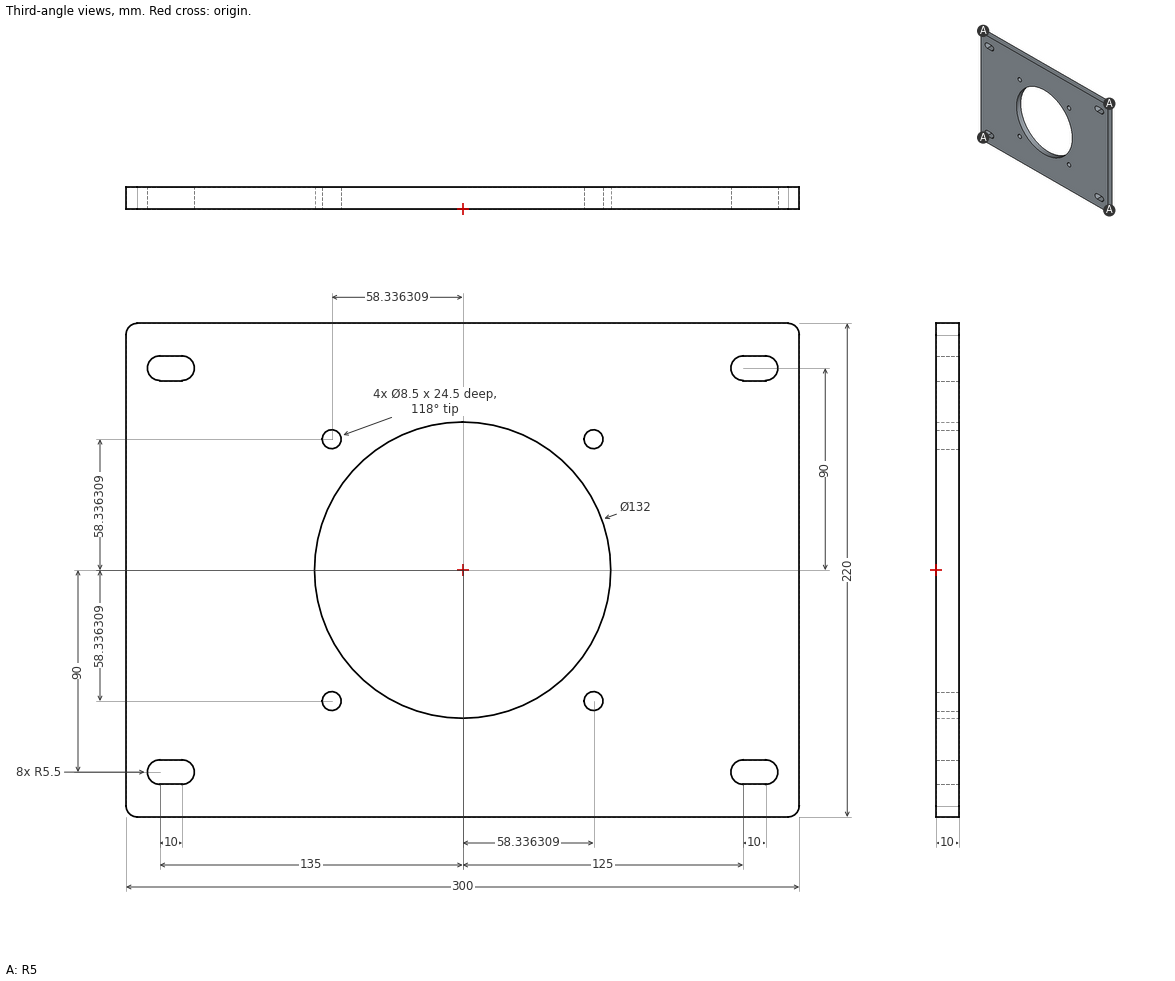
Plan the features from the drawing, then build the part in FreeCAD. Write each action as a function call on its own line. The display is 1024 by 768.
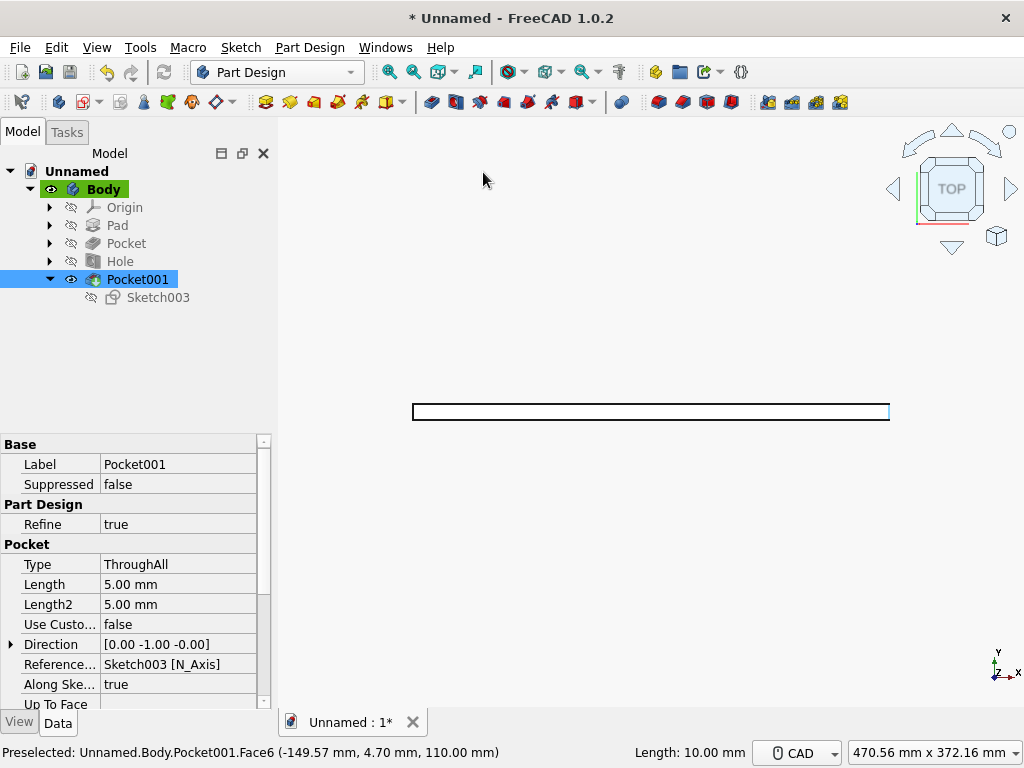
click(413, 411, ctrl)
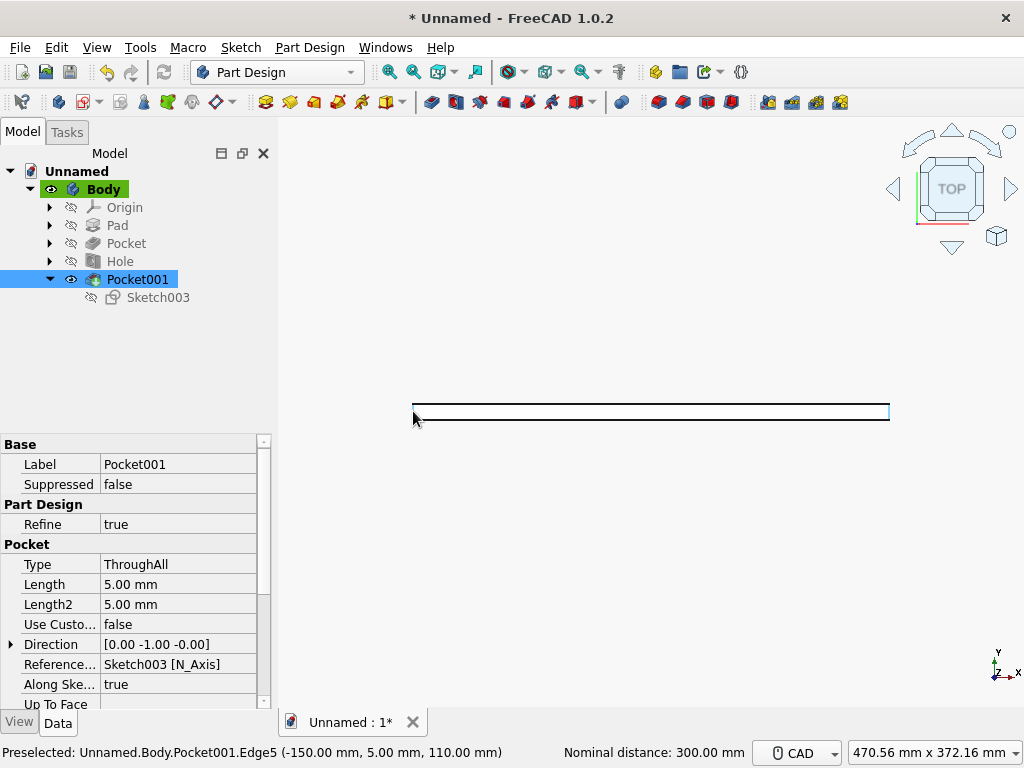
scroll(413, 411, up, 5)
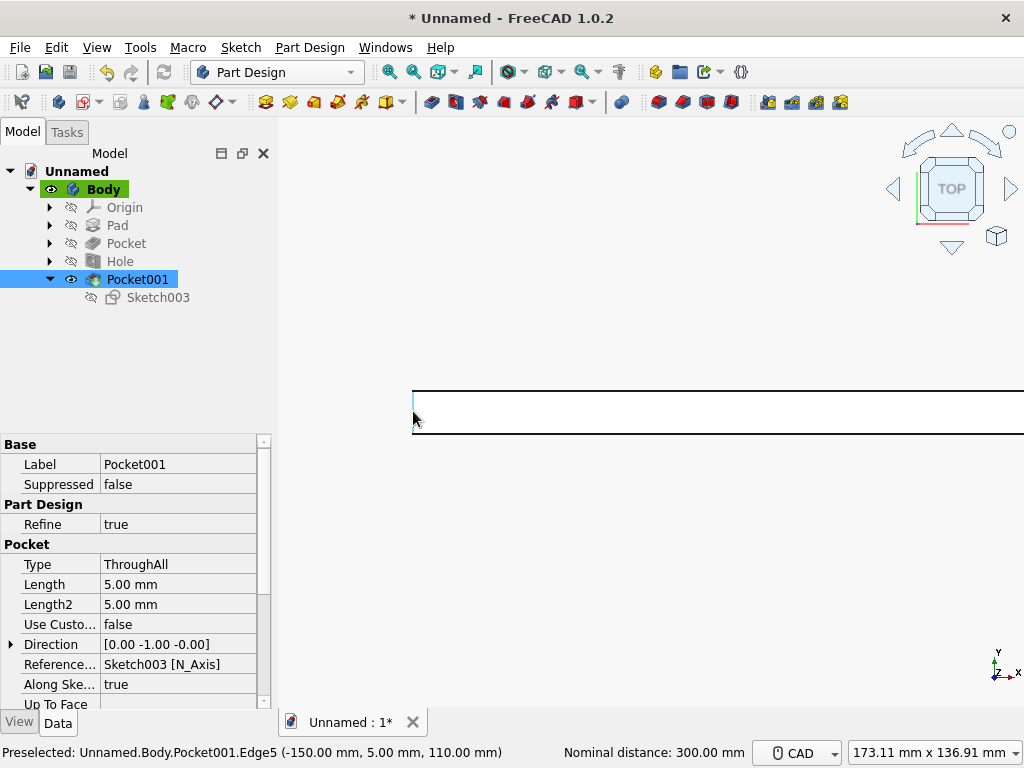
key(v)
key(f)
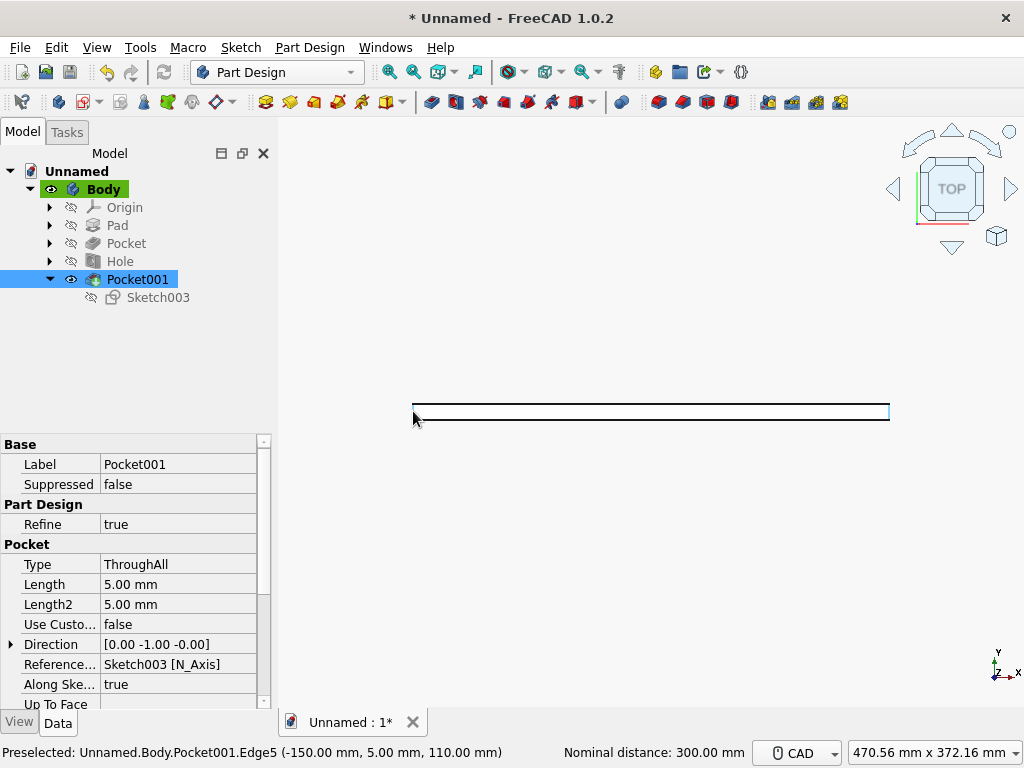
key(1)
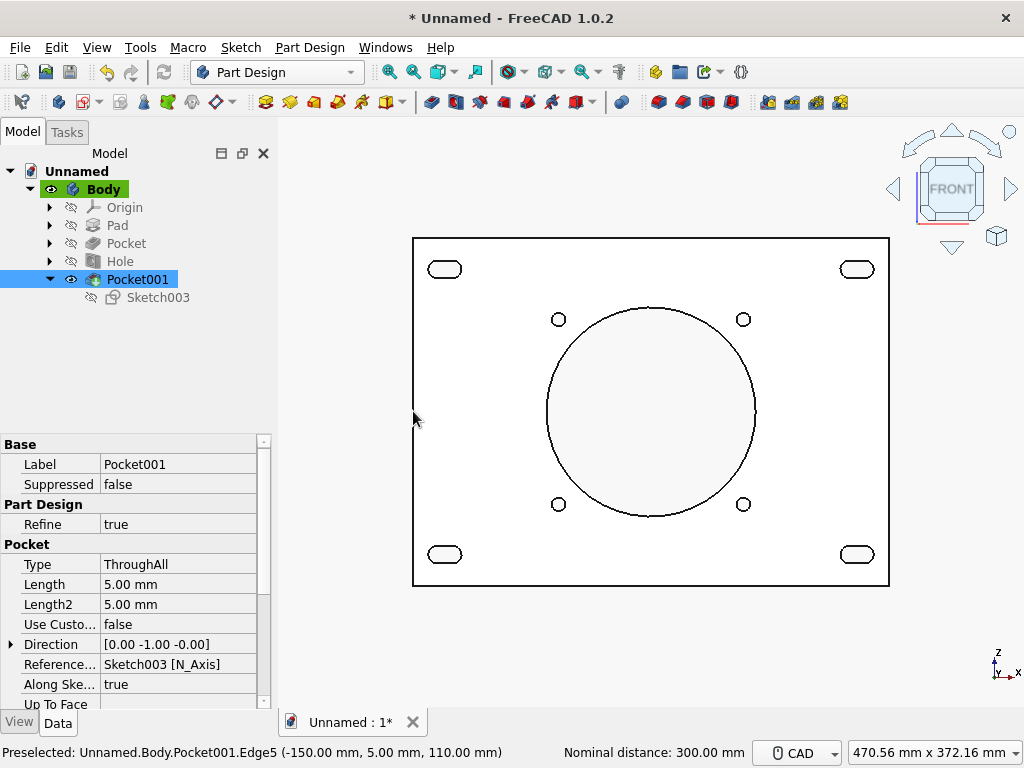
scroll(413, 585, up, 5)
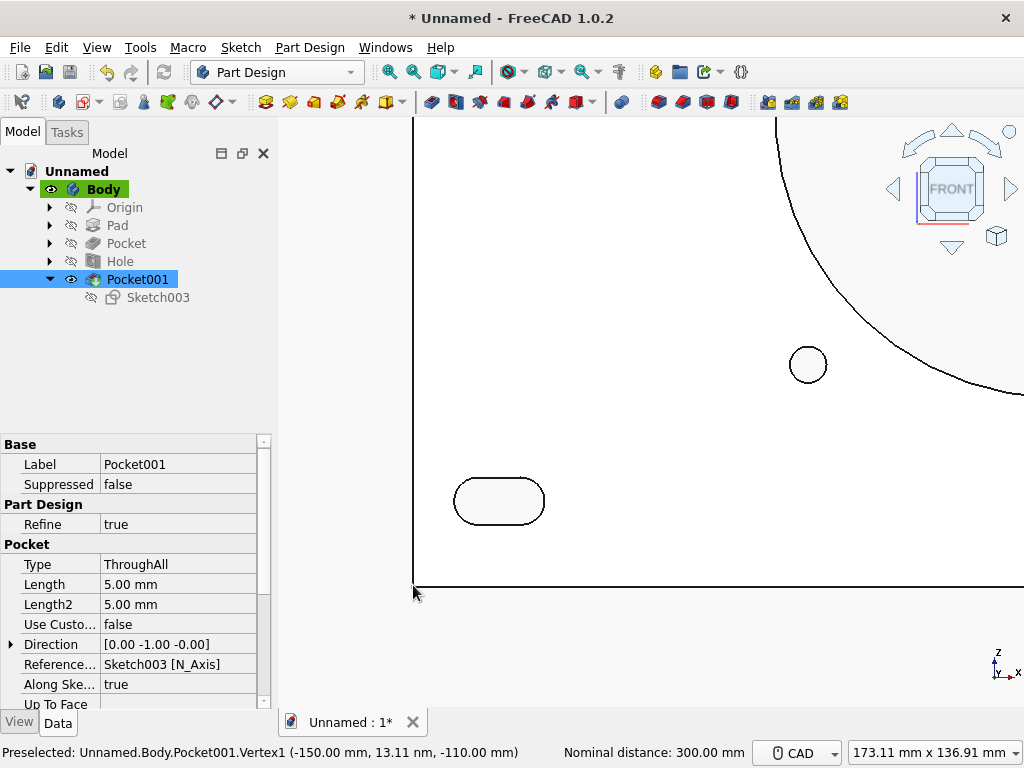
click(390, 72)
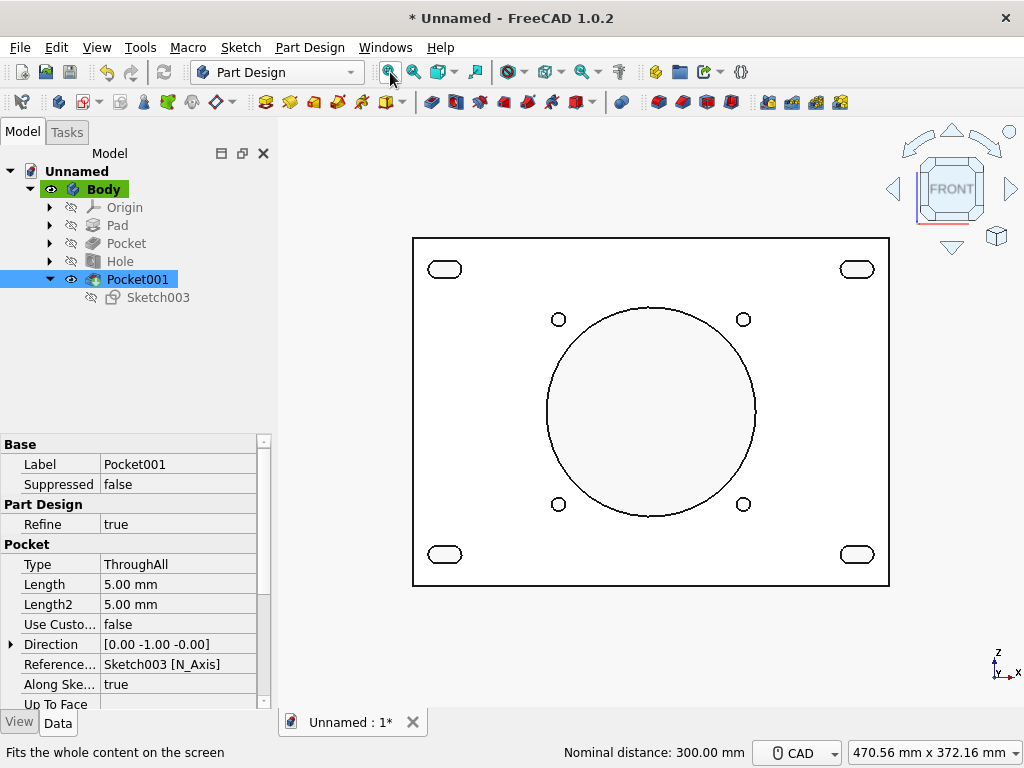
key(3)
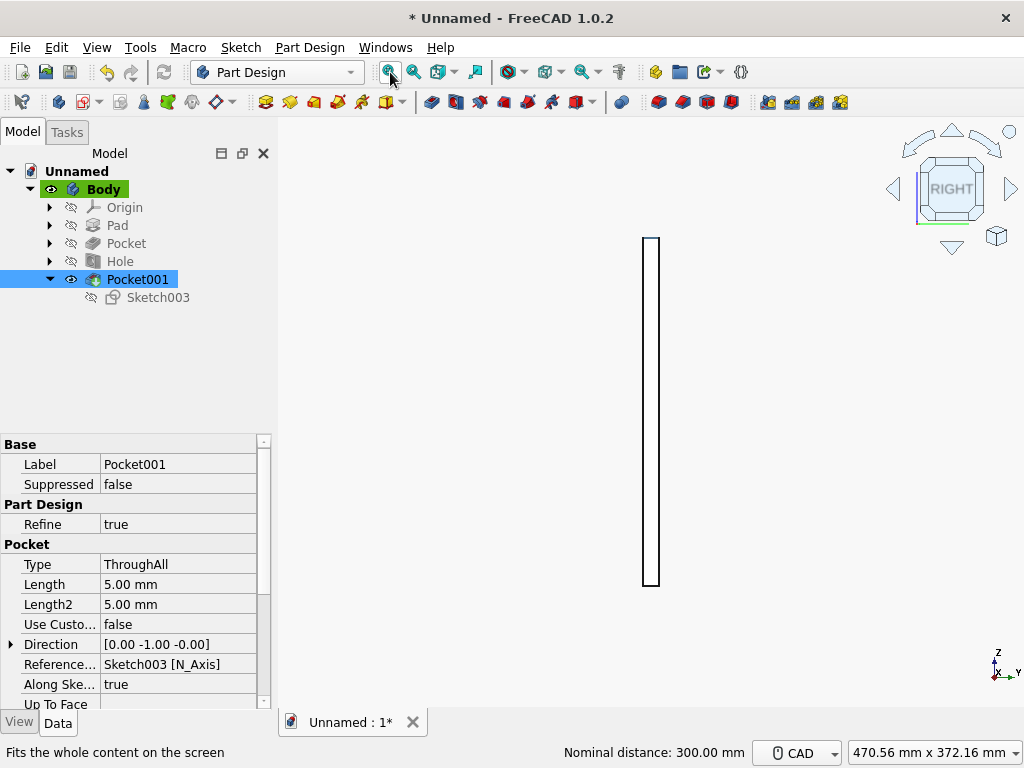
click(651, 585, ctrl)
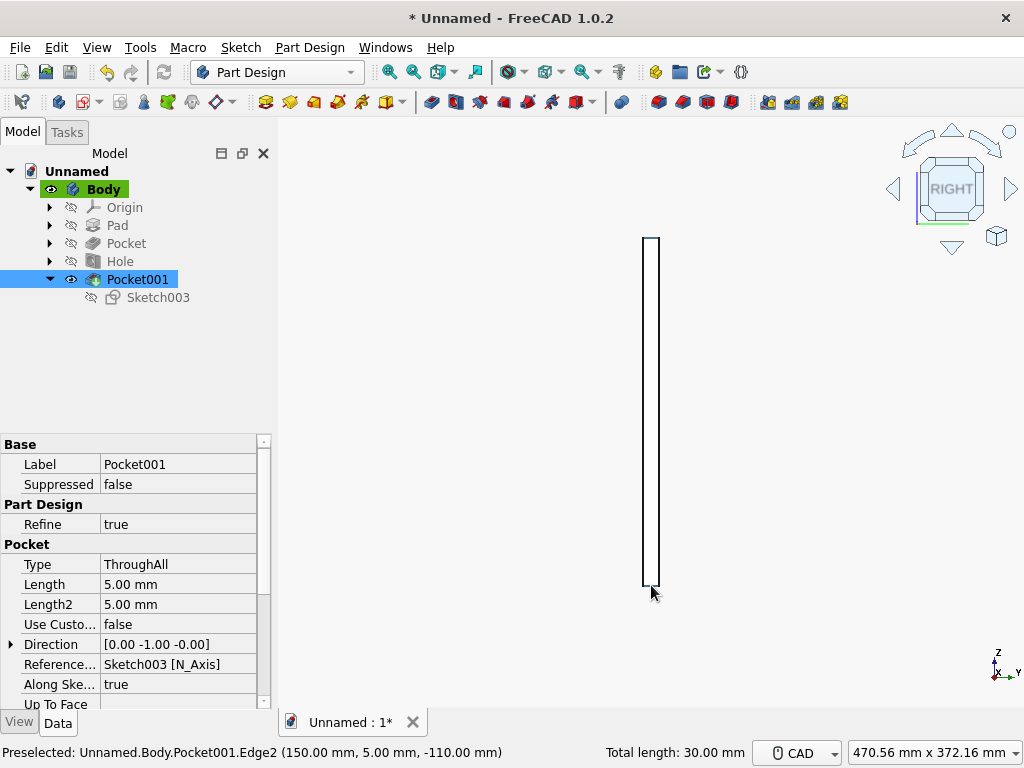
scroll(651, 585, up, 5)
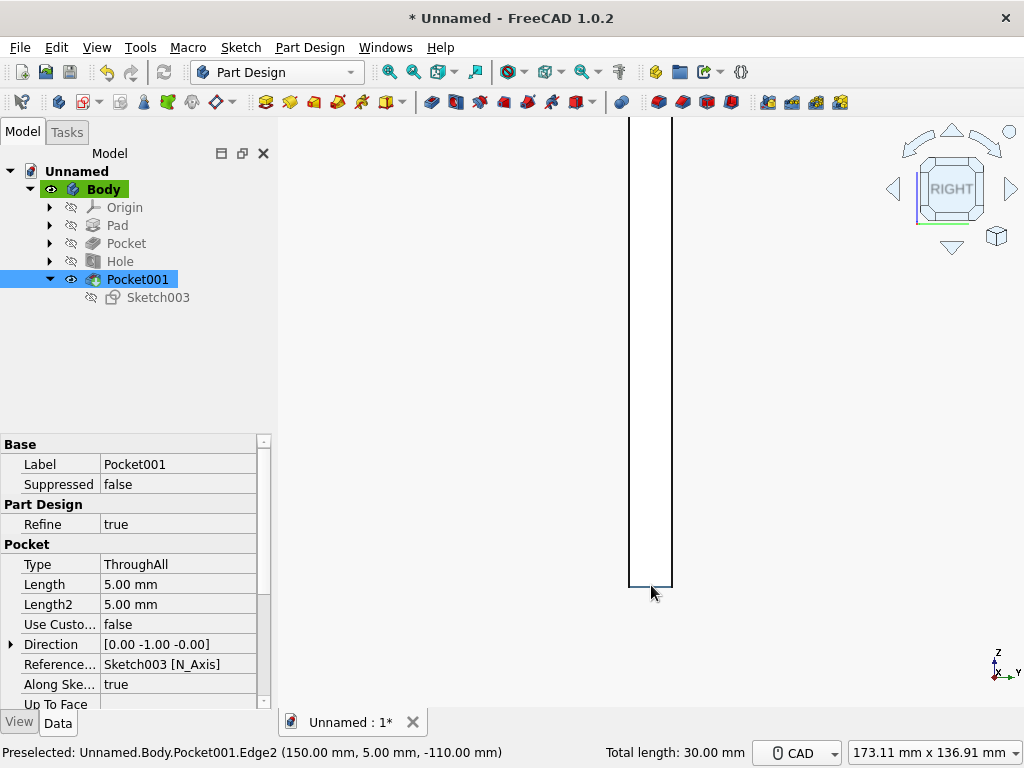
click(390, 72)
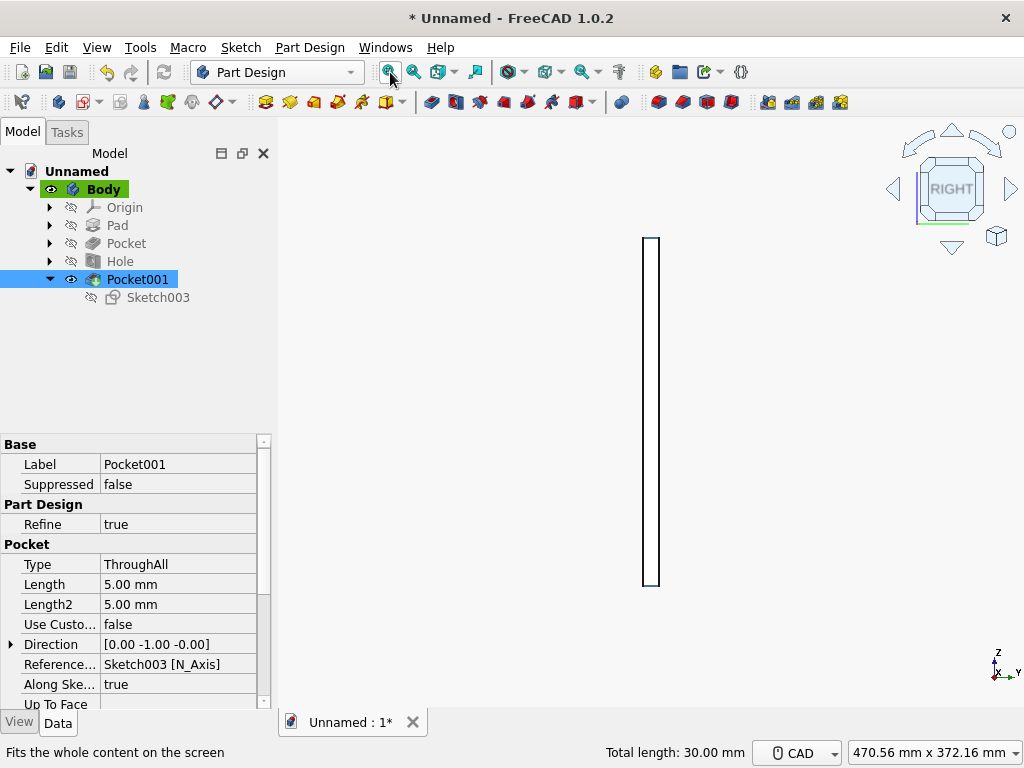
key(5)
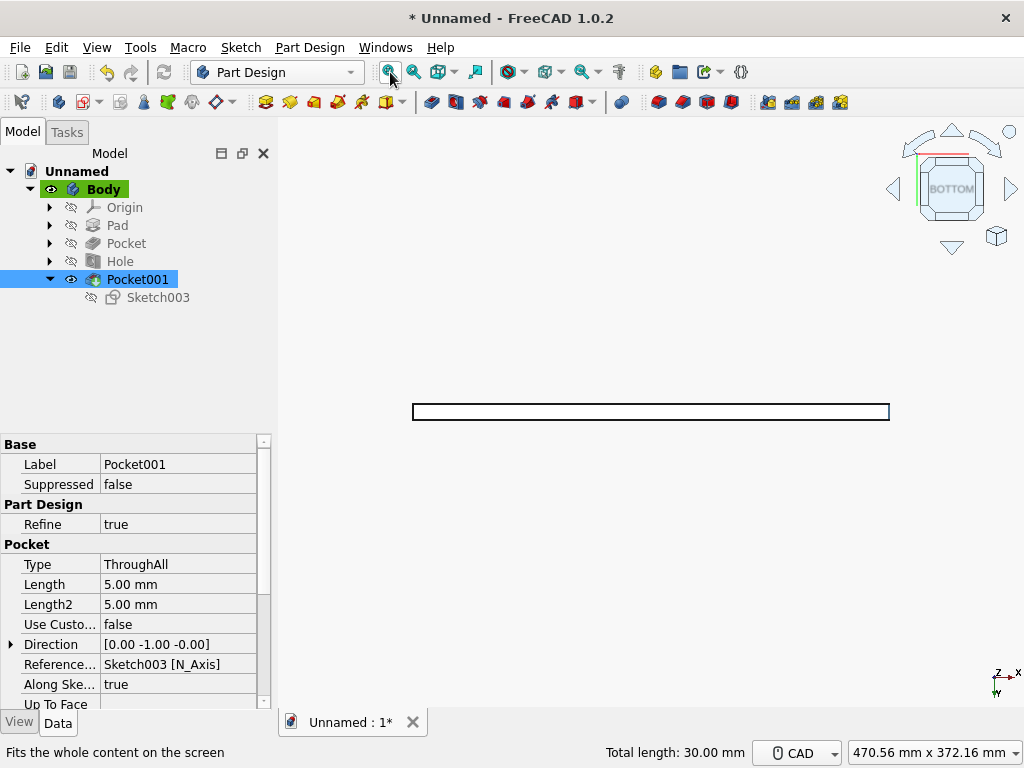
click(413, 411, ctrl)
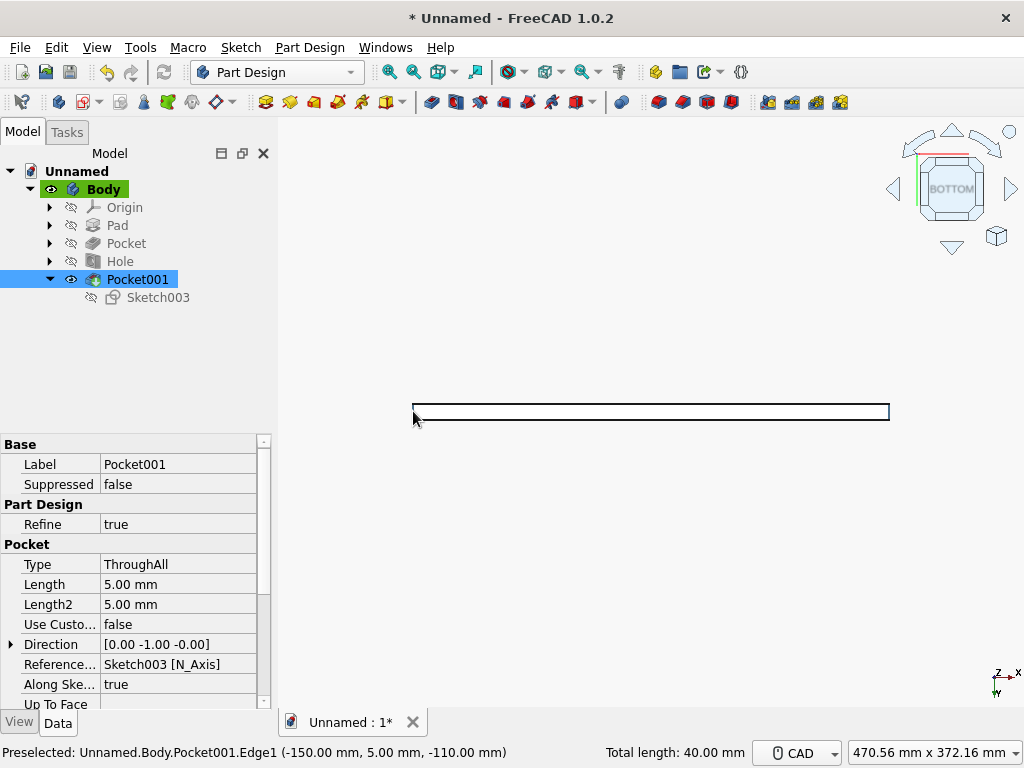
click(660, 102)